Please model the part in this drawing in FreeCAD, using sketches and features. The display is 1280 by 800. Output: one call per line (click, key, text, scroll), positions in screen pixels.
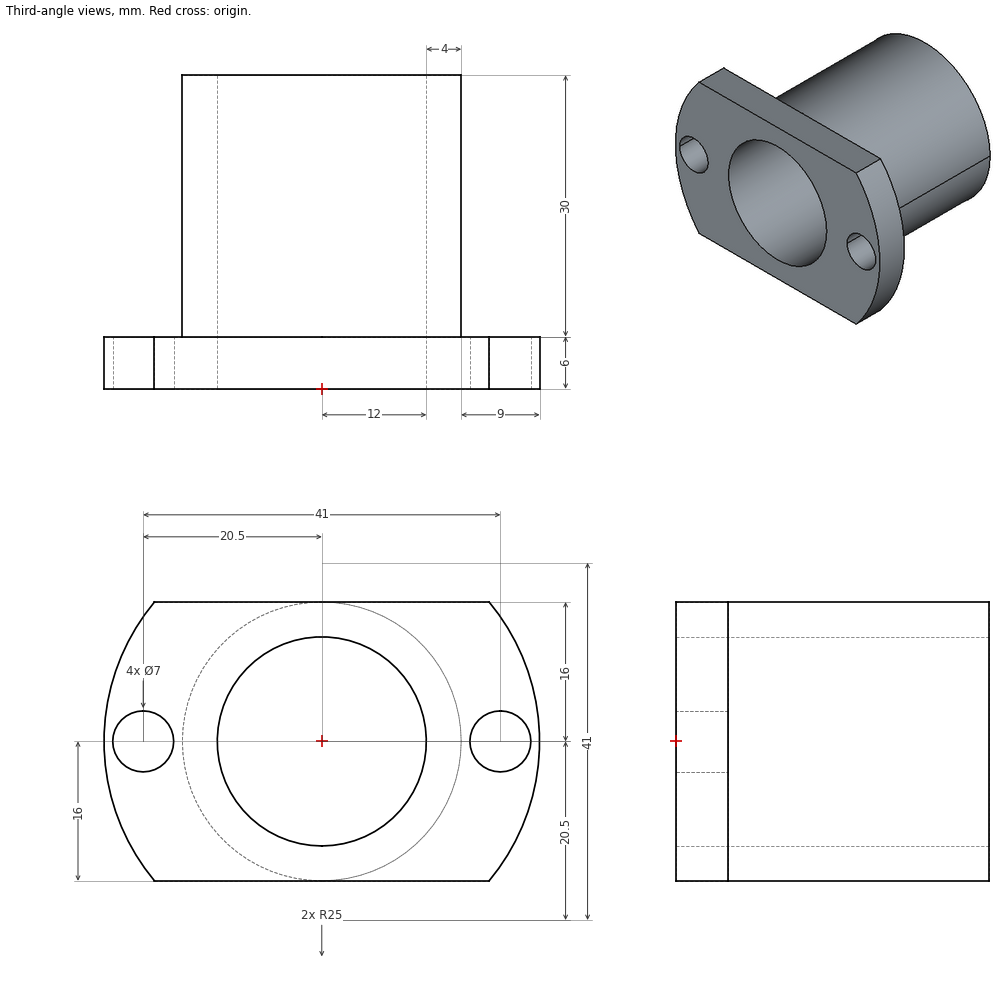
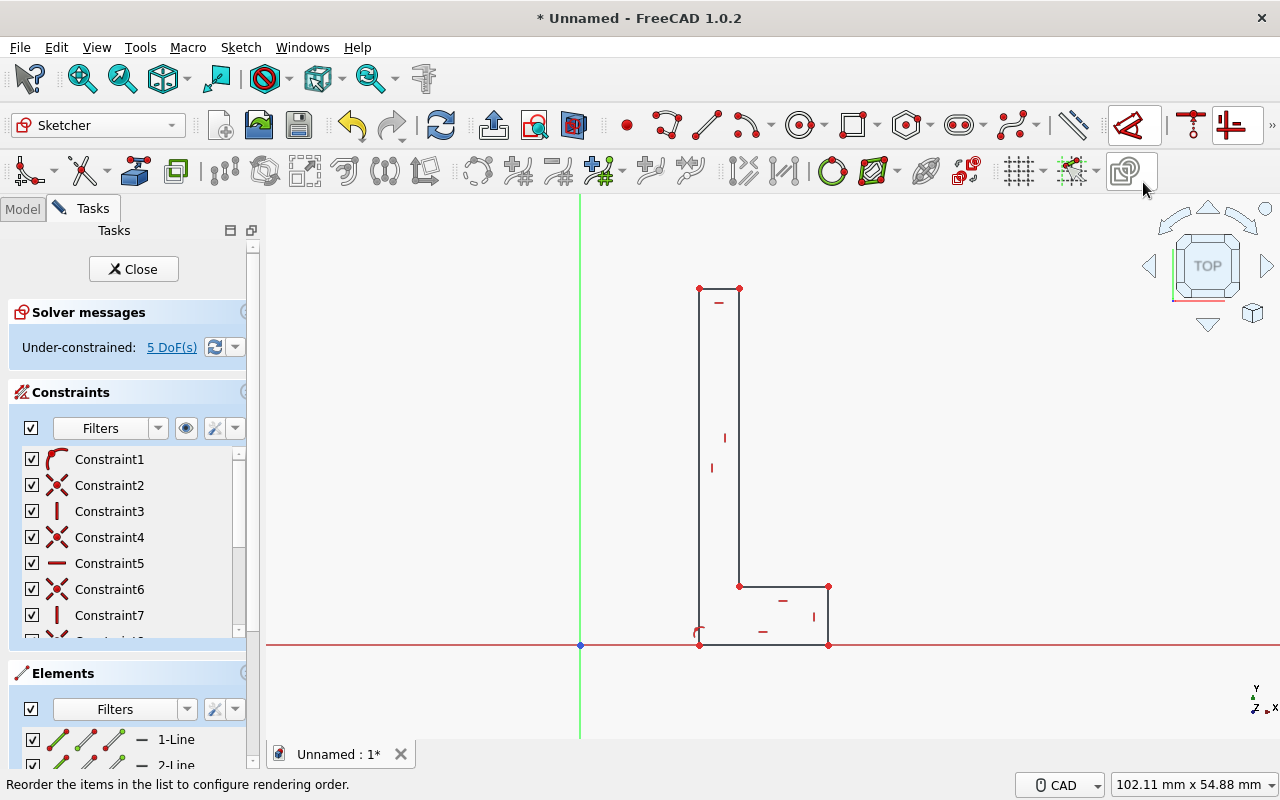
click(828, 628)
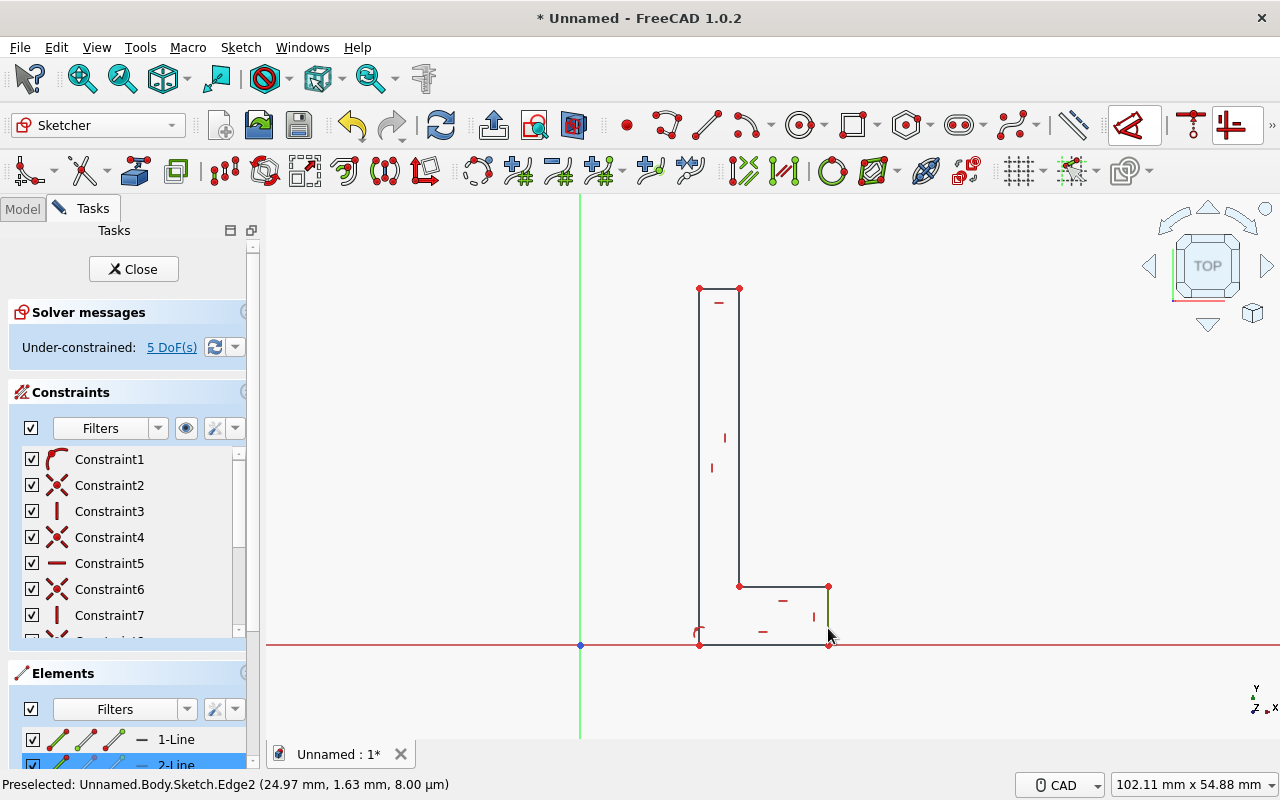
click(1156, 126)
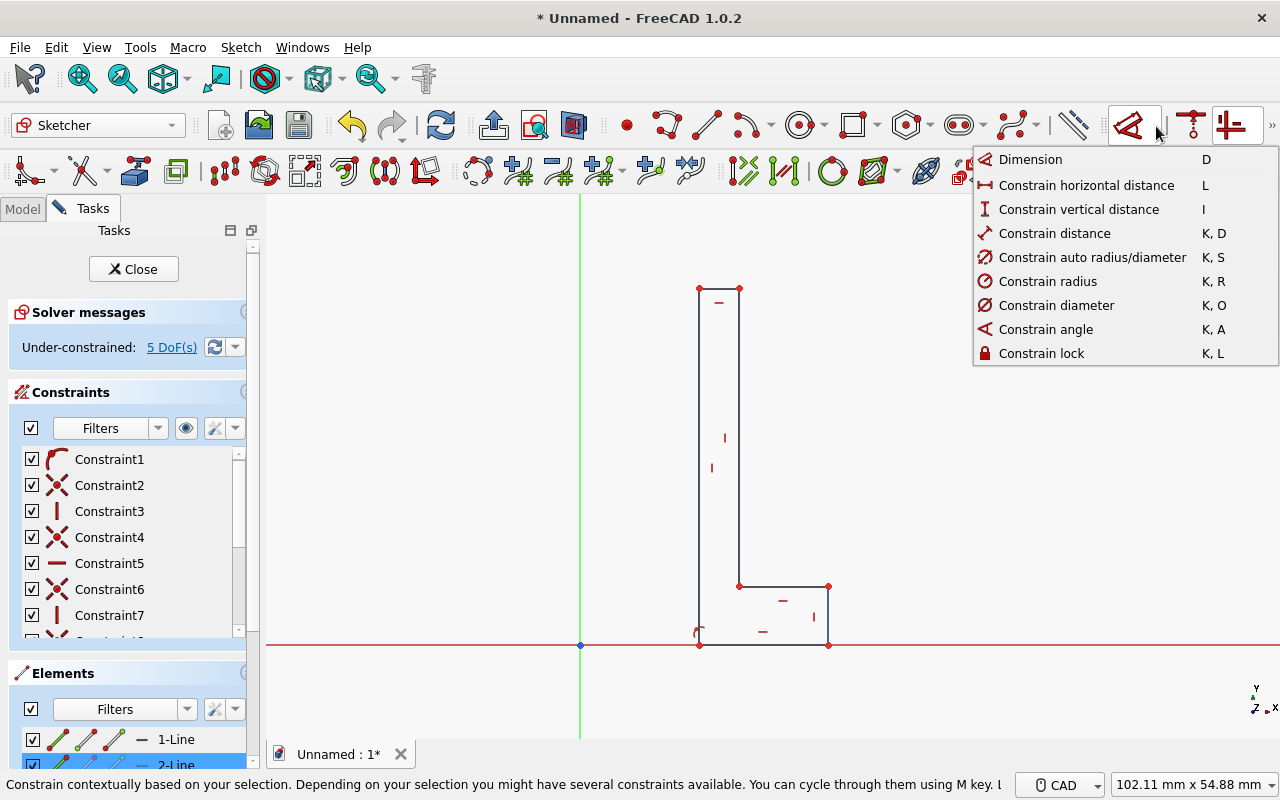
click(1126, 209)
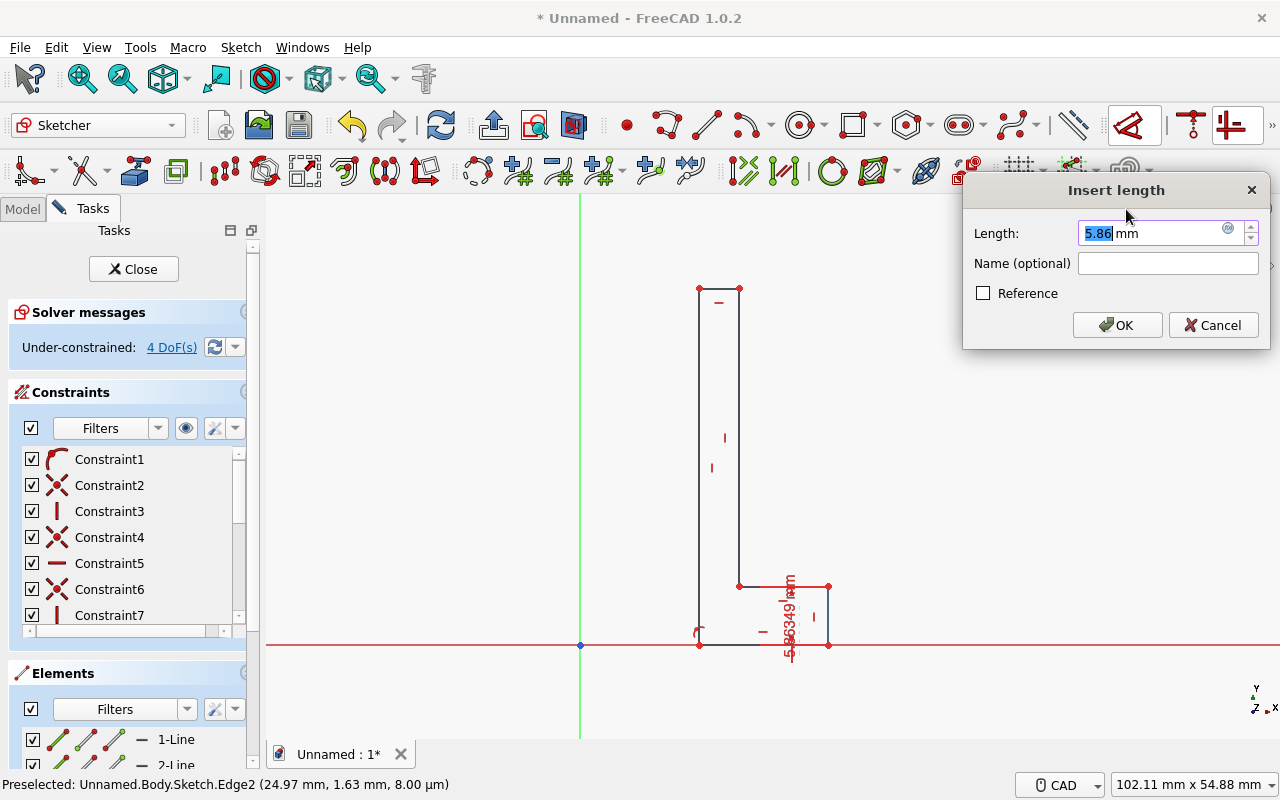
text(6)
key(Return)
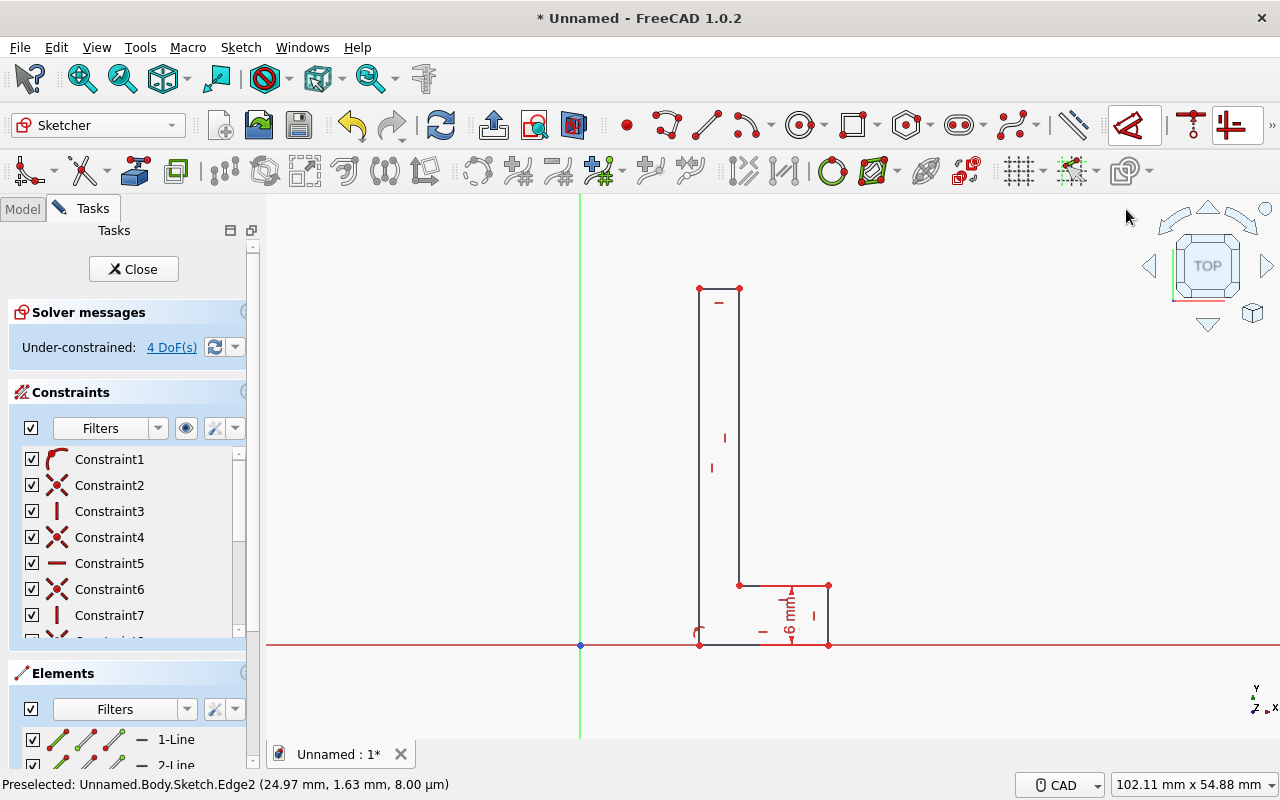
click(801, 586)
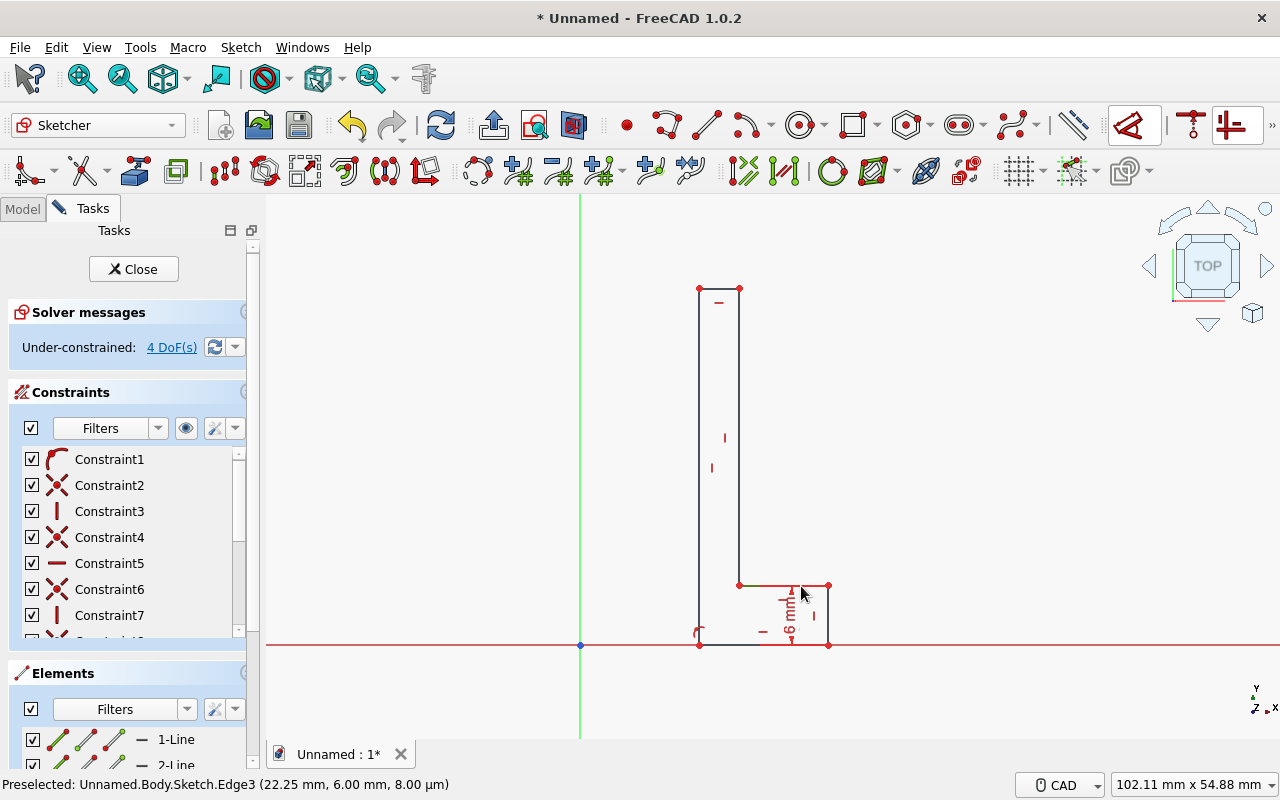
click(1156, 126)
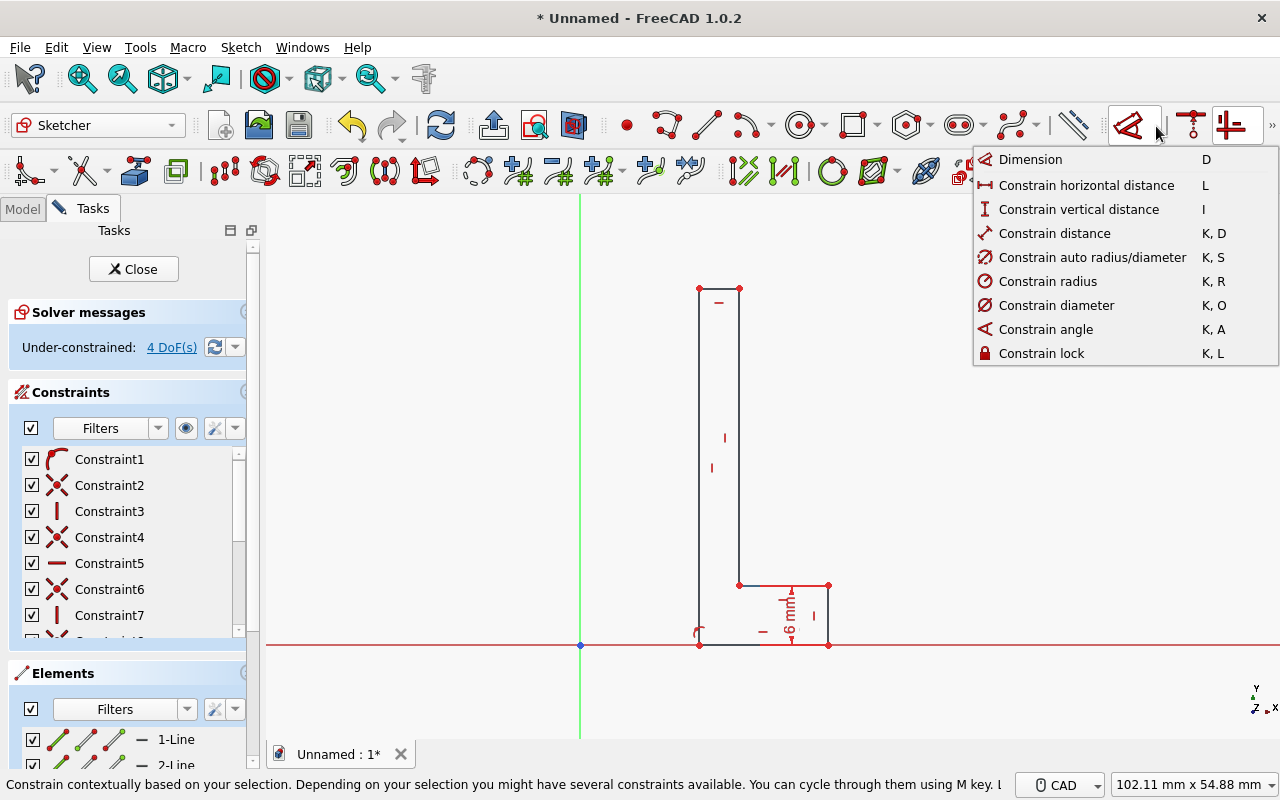
click(1126, 185)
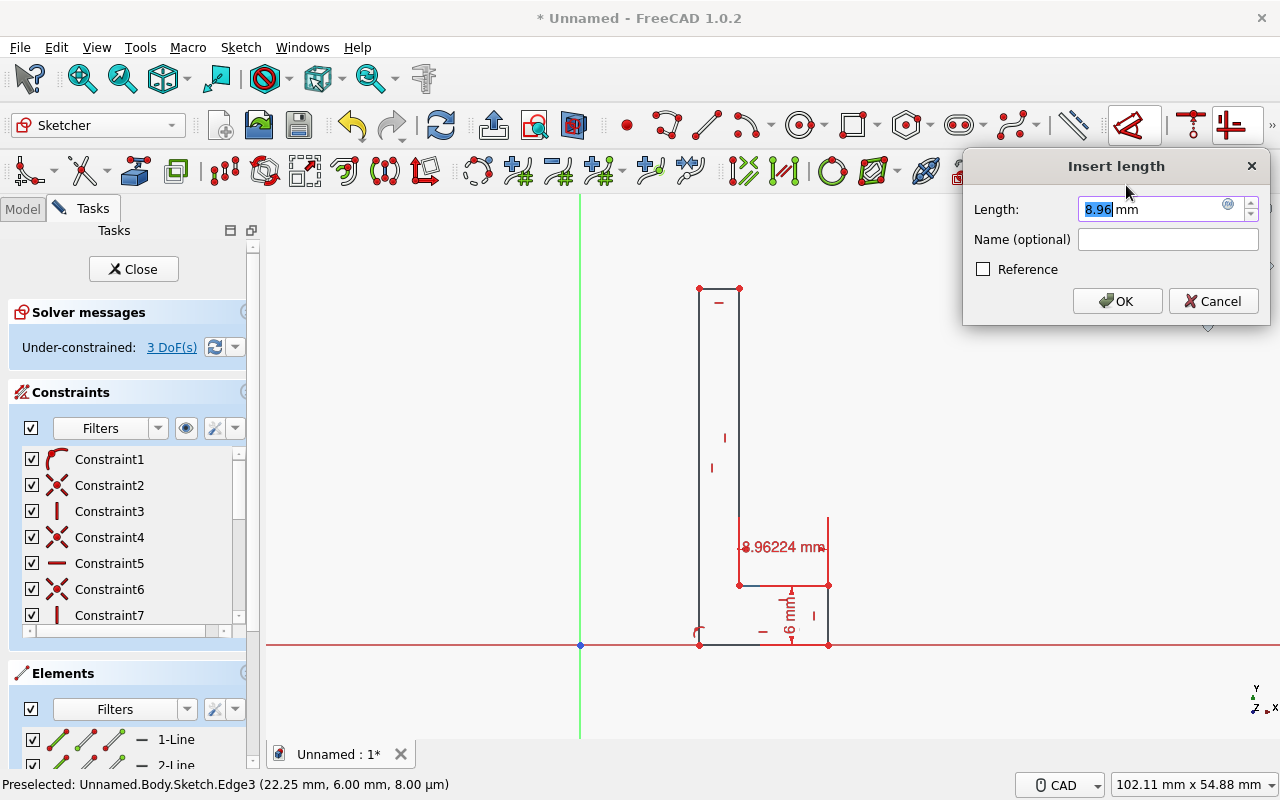
text(9)
key(Return)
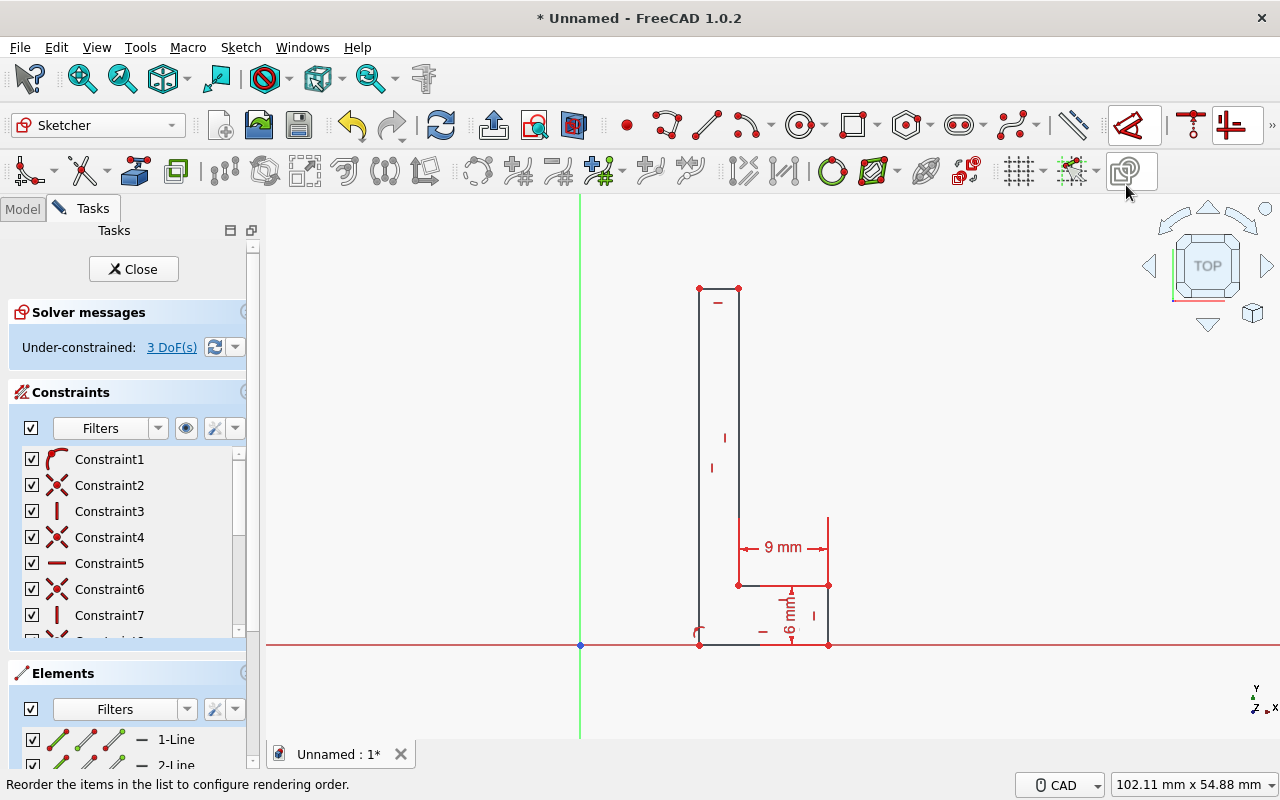
click(727, 289)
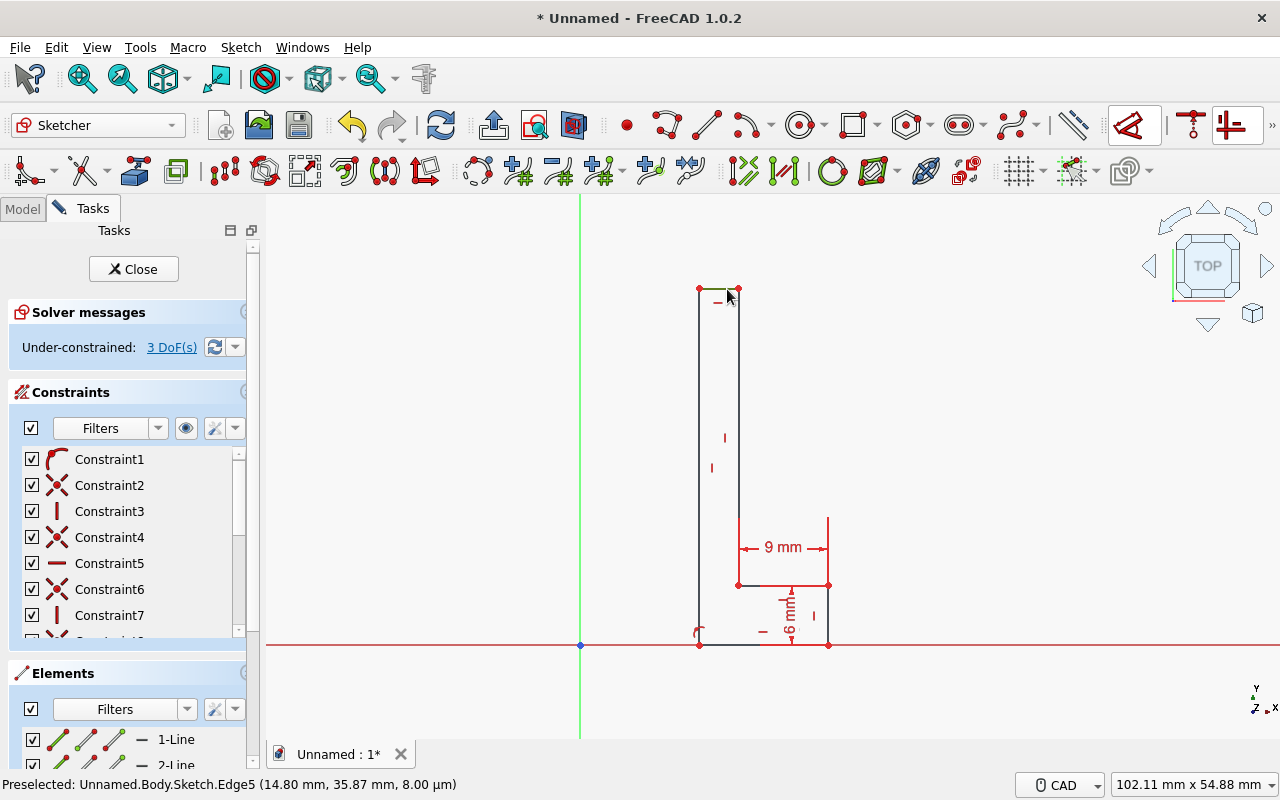
click(1156, 126)